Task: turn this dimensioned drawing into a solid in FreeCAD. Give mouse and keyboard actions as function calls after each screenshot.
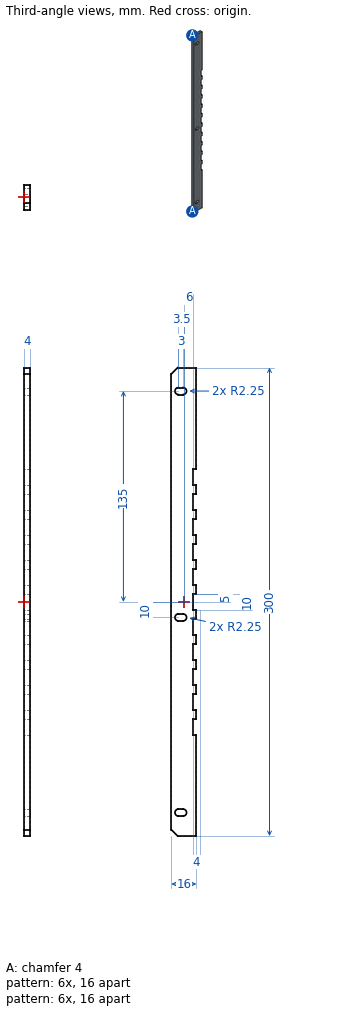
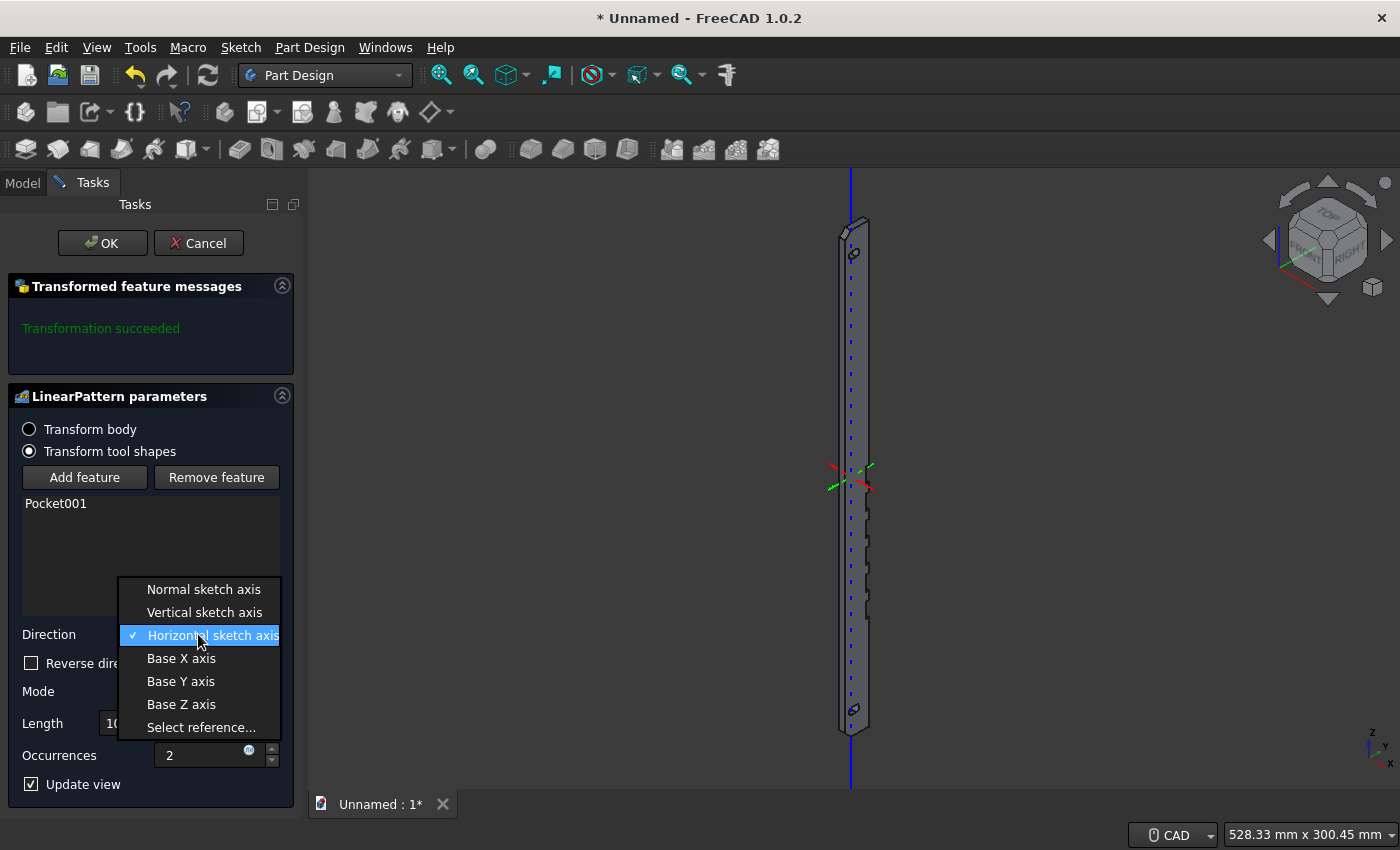
click(198, 704)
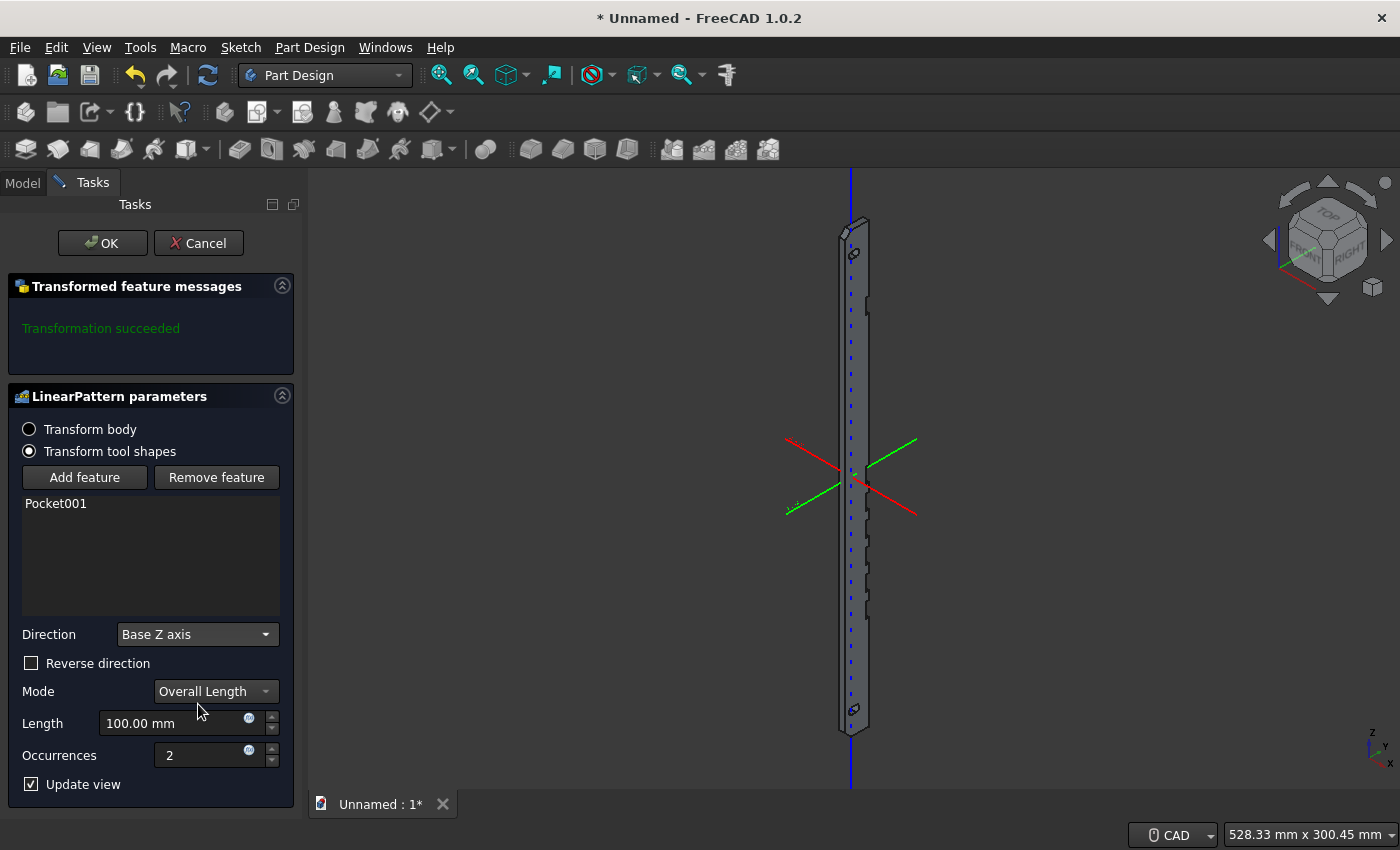
click(217, 692)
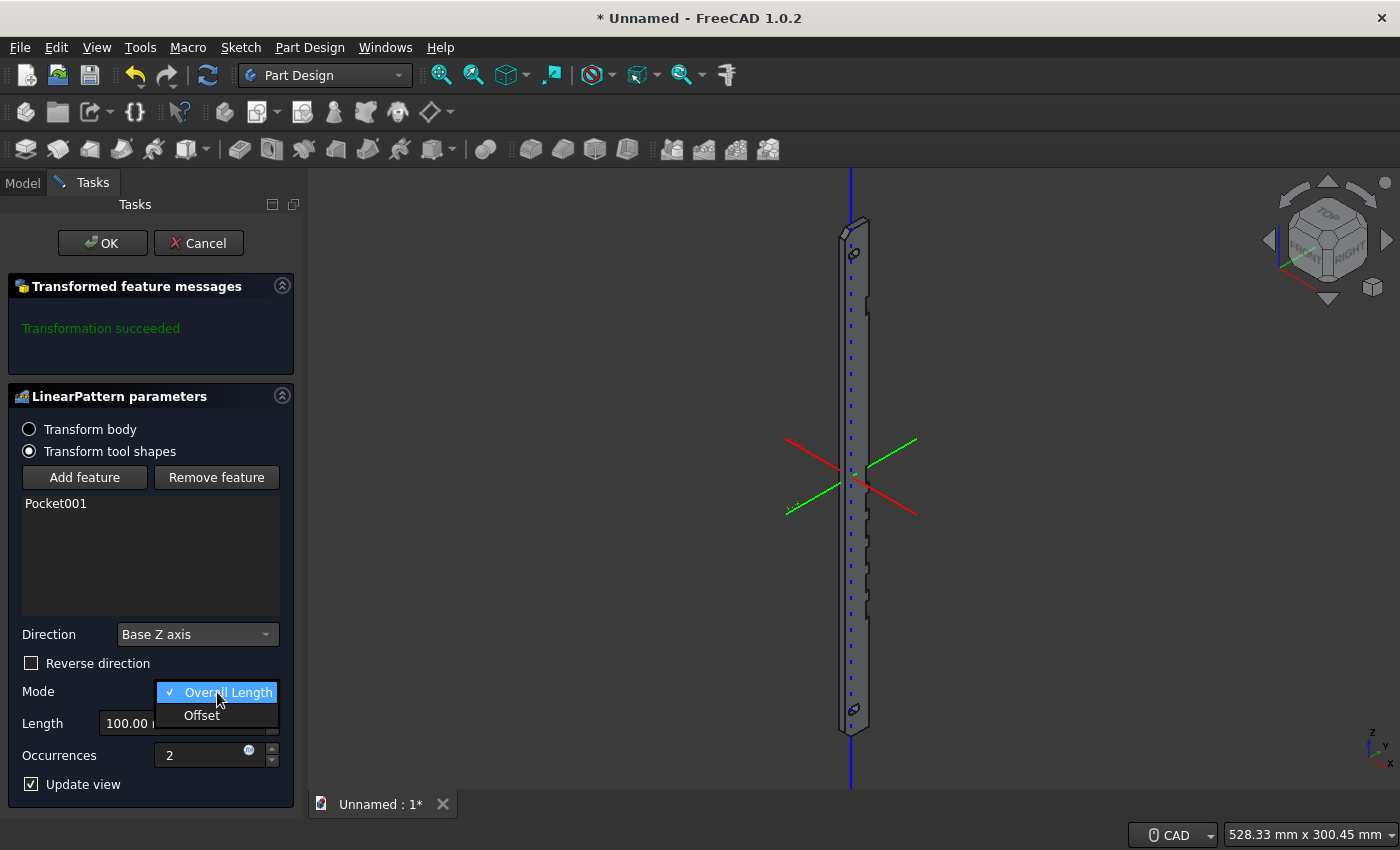
click(216, 716)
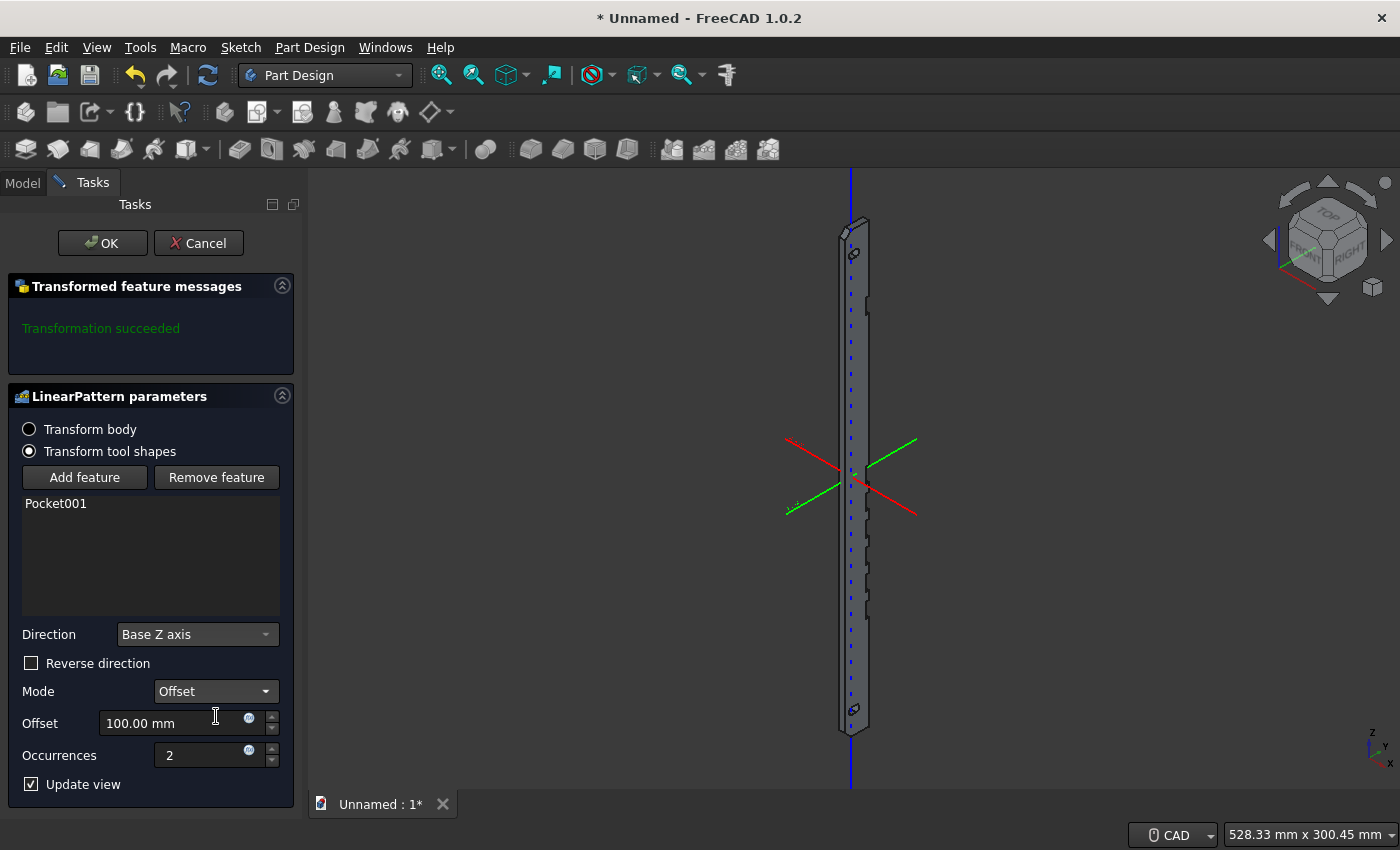
triple_click(182, 723)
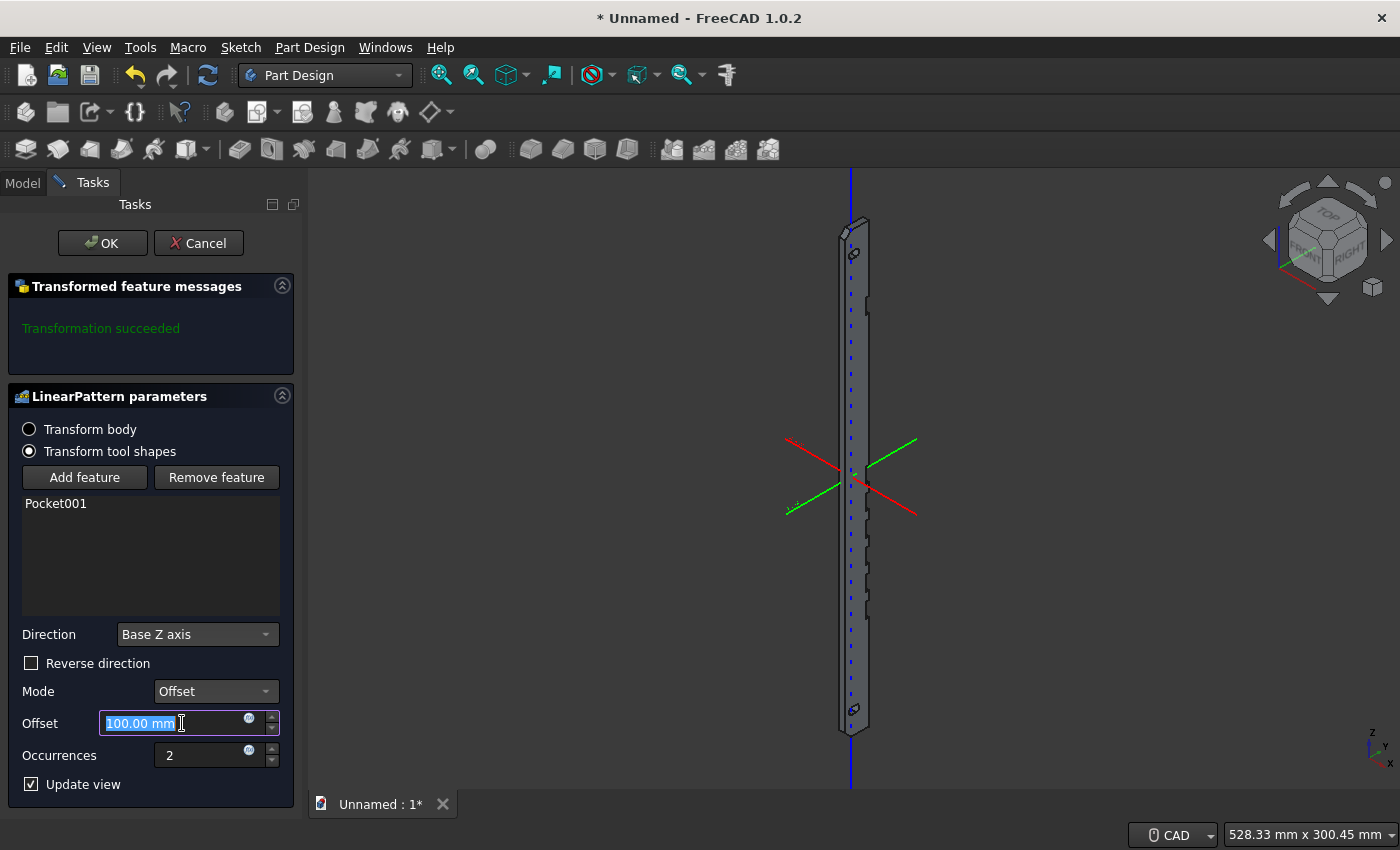
text(16)
key(Tab)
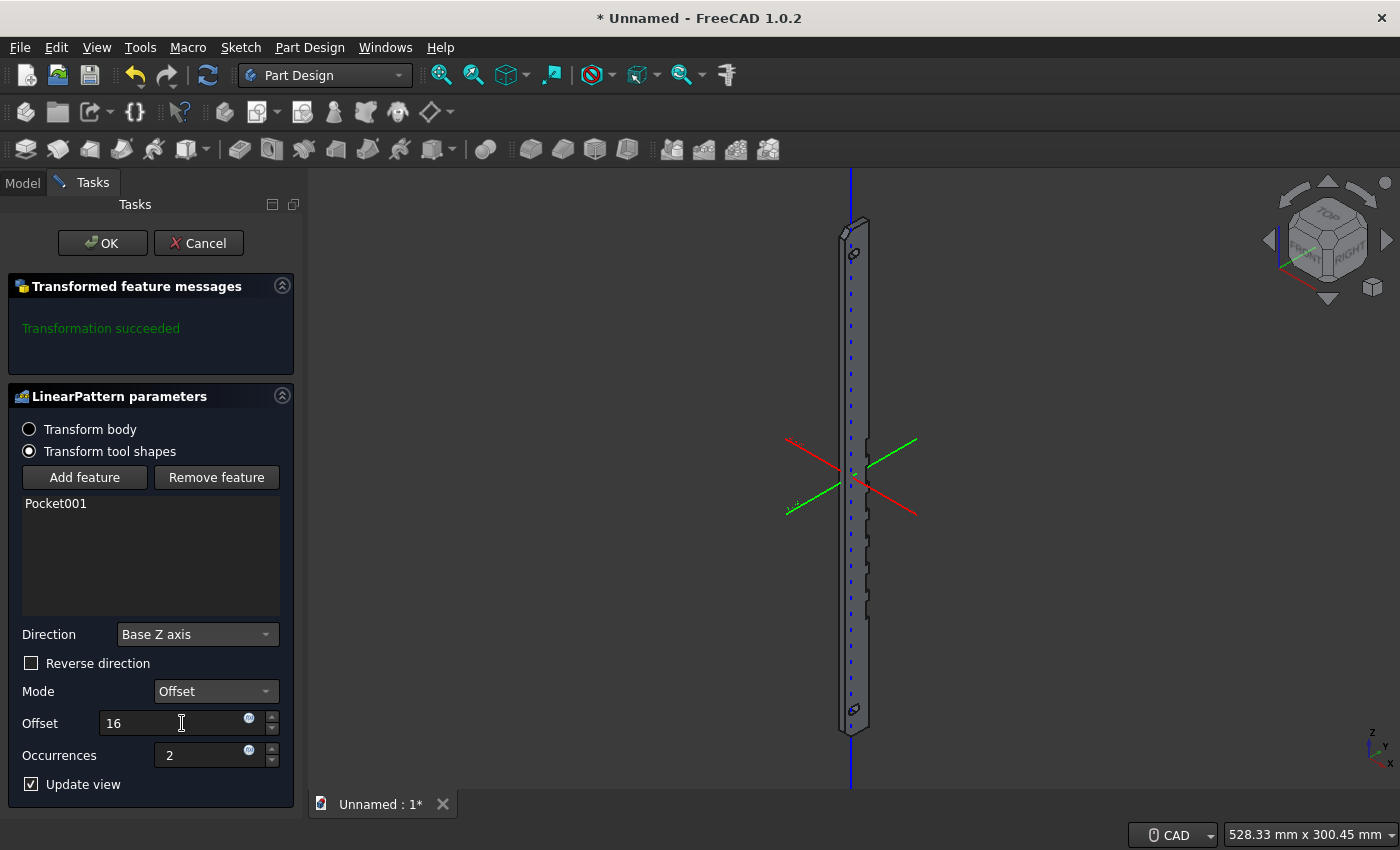
triple_click(209, 755)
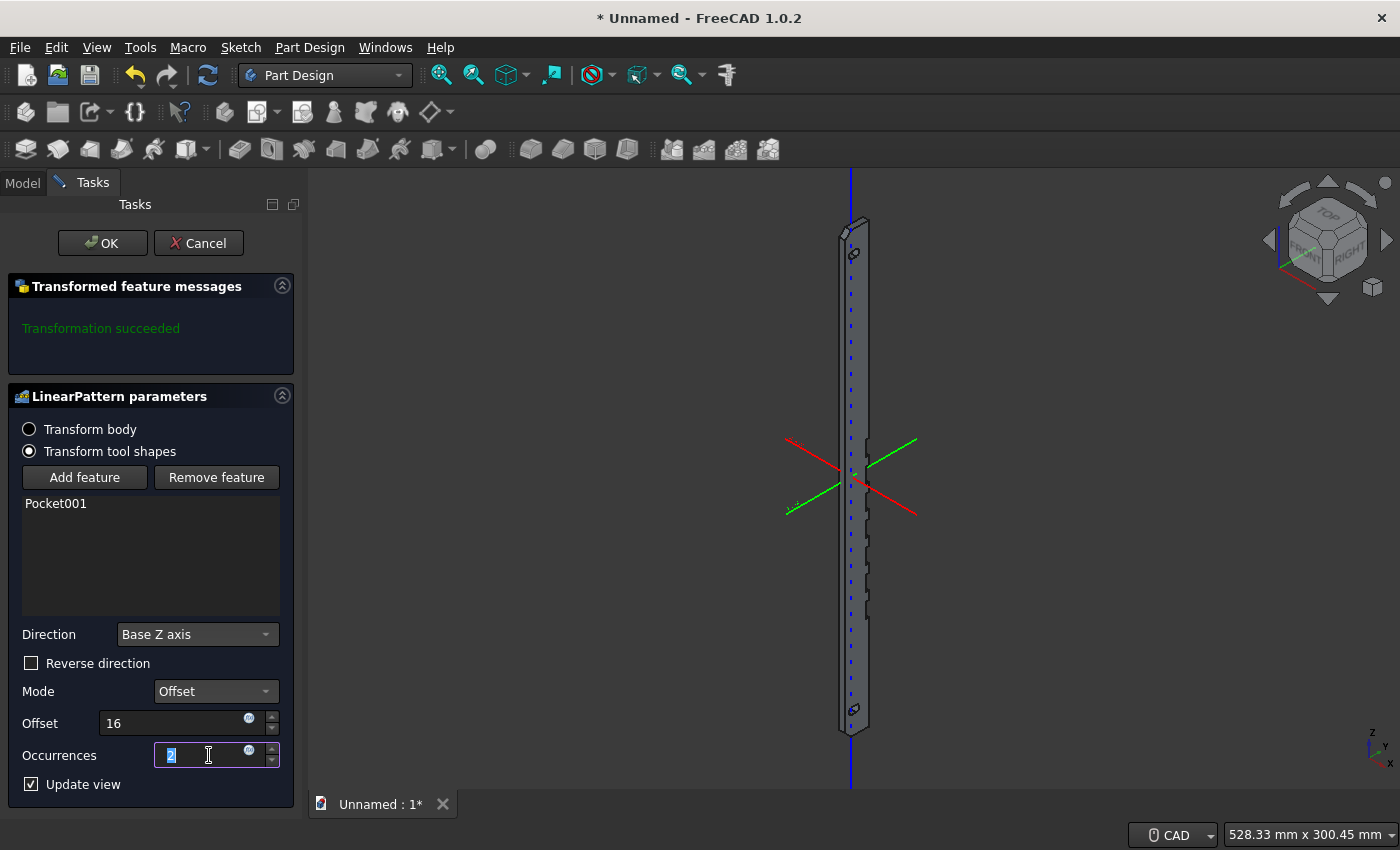
text(6)
key(Tab)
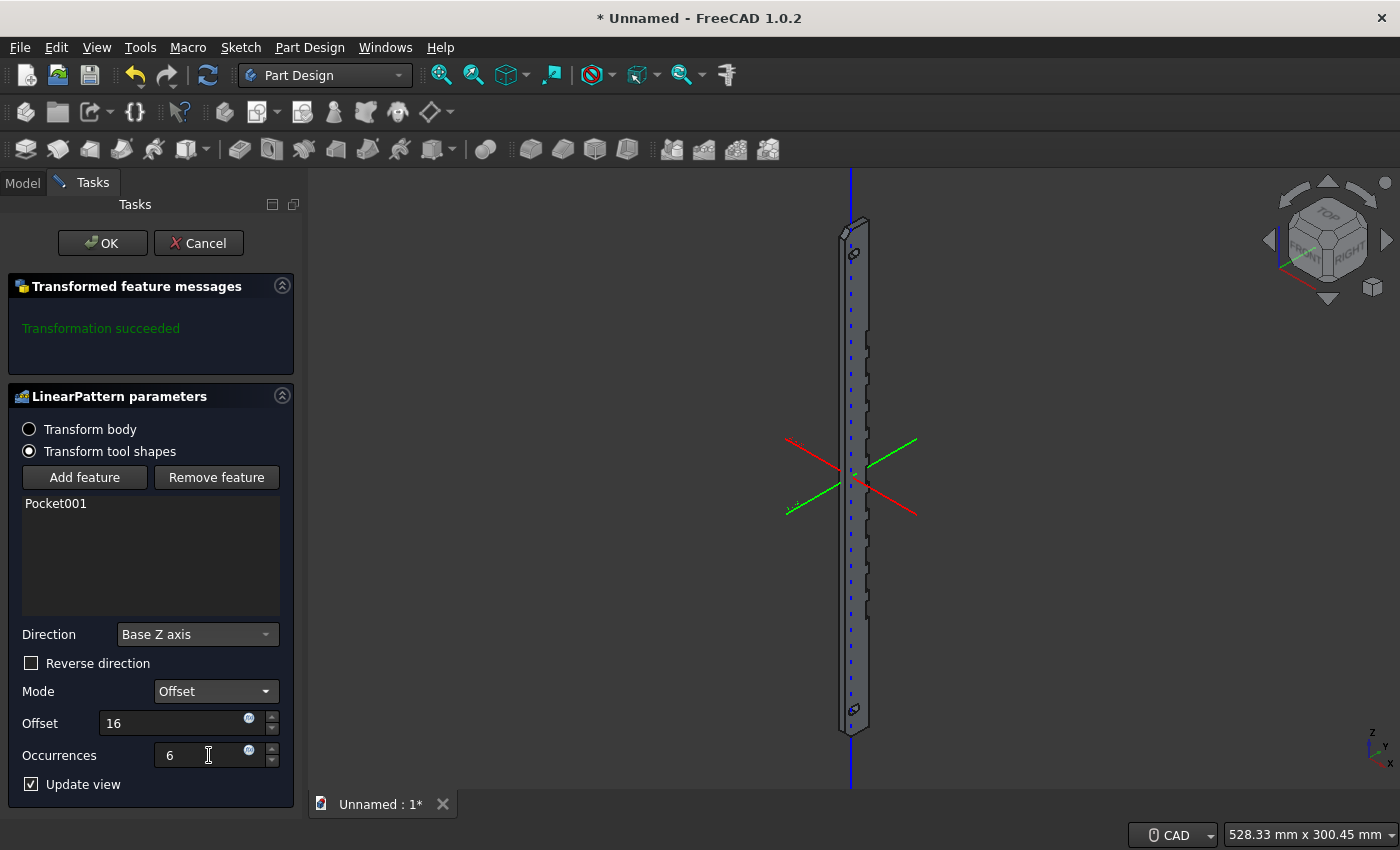
click(103, 243)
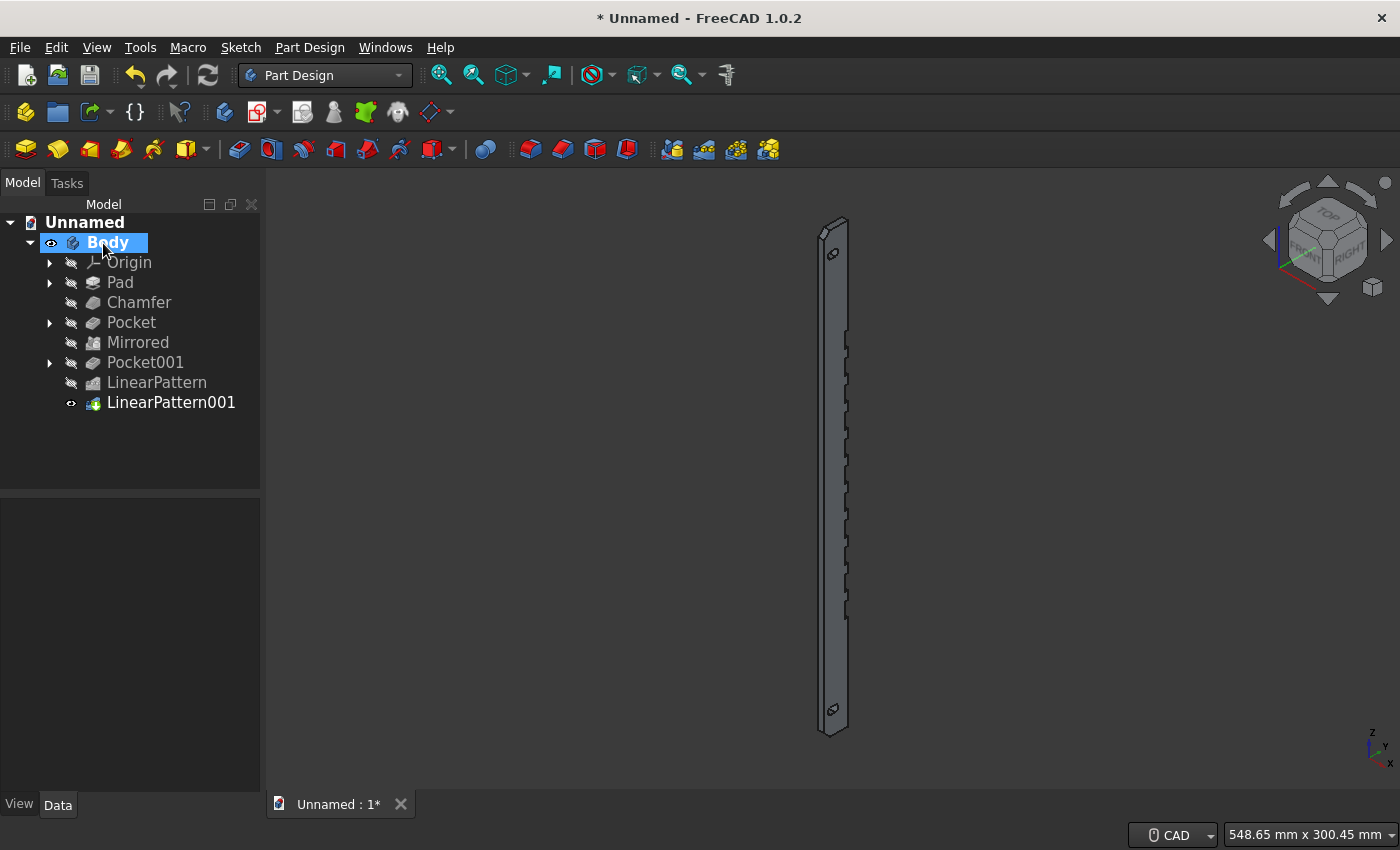
click(836, 624)